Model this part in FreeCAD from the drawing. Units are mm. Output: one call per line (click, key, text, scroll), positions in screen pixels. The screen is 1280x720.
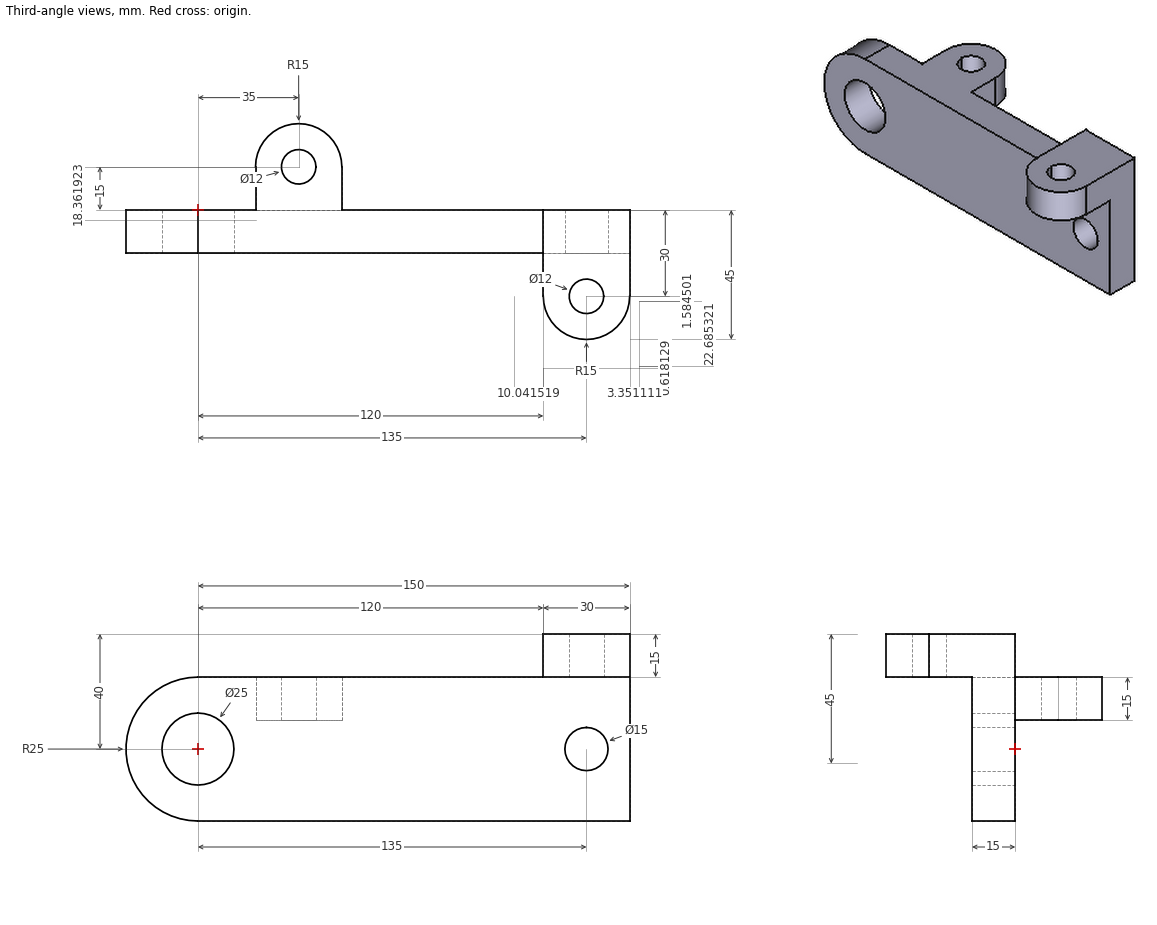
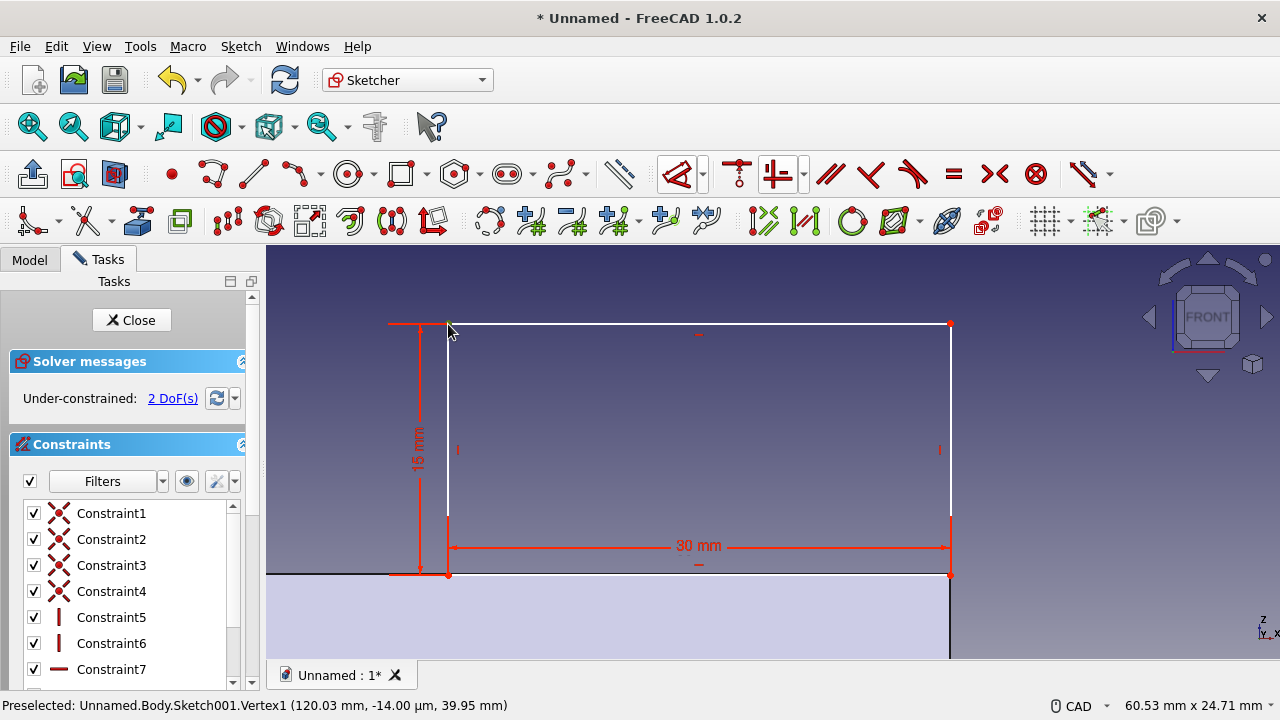
key(i)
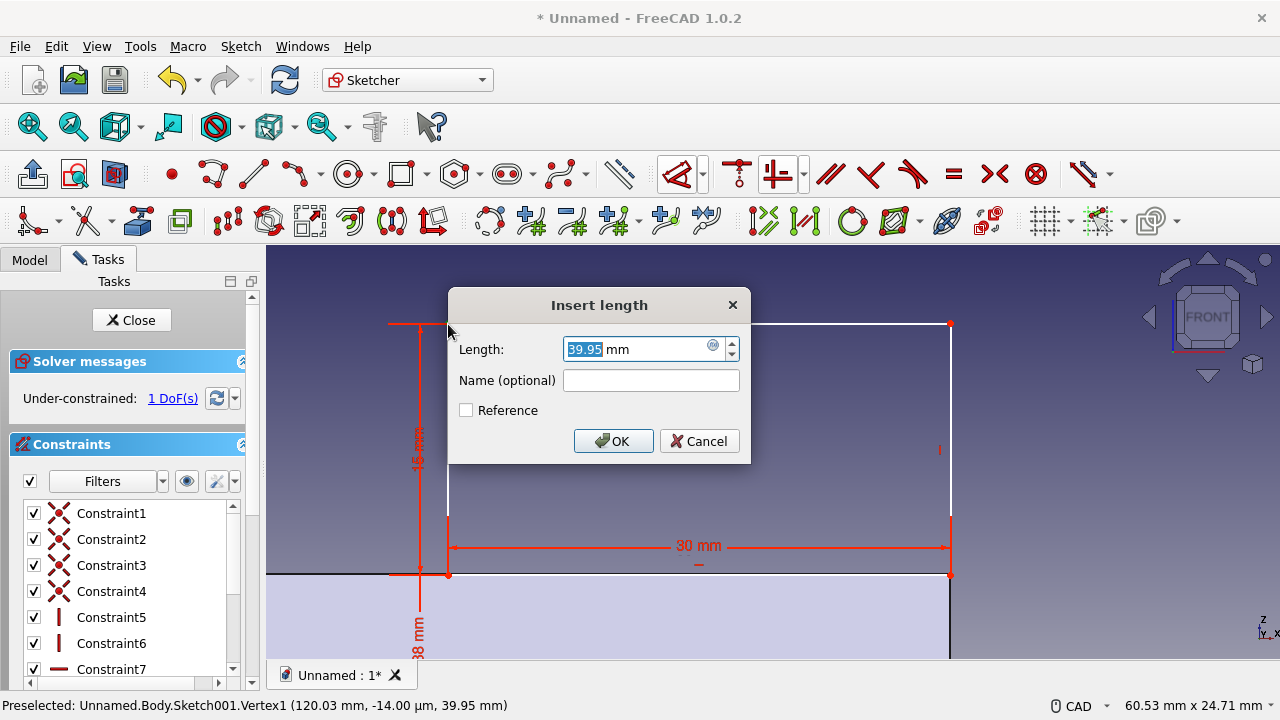
text(40)
key(Return)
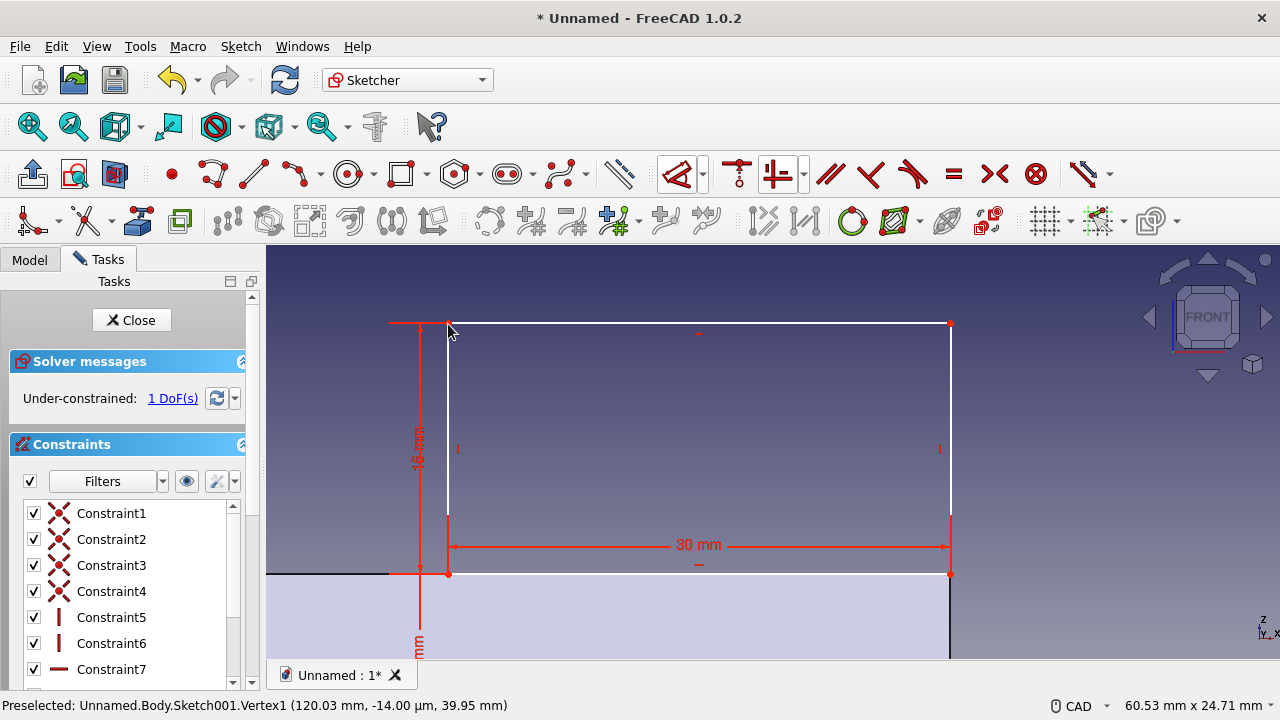
click(448, 323)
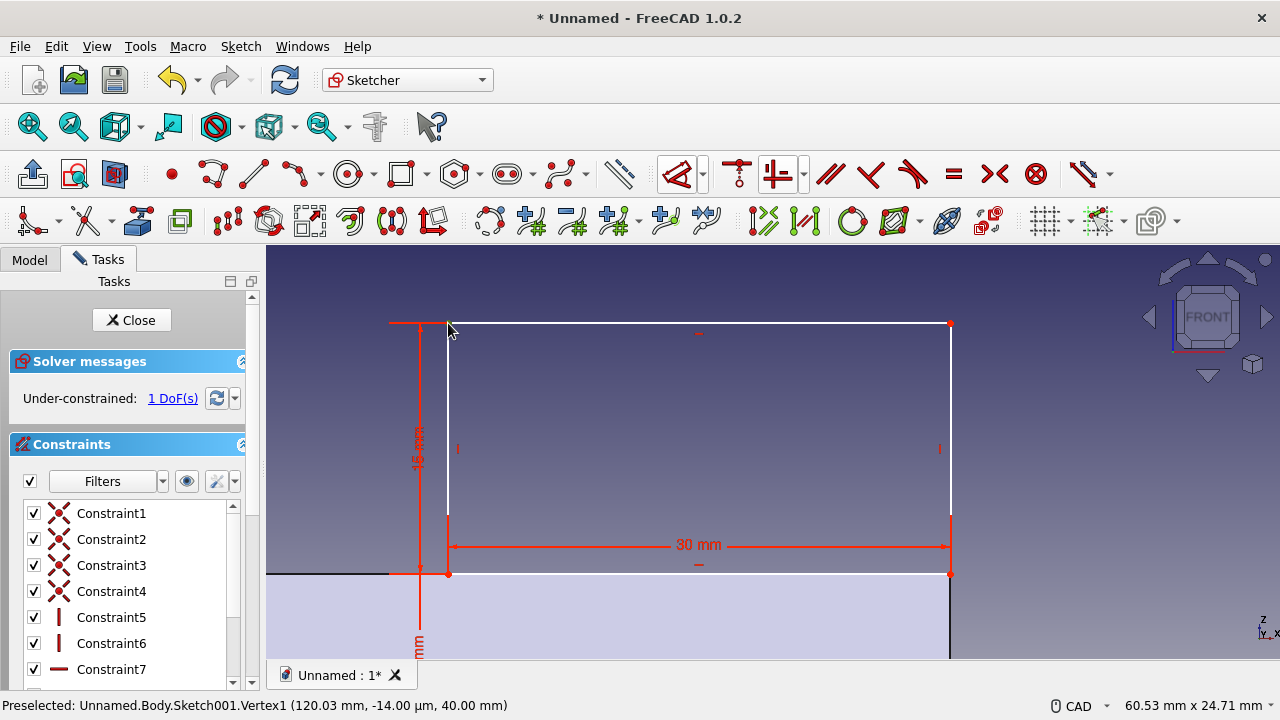
key(l)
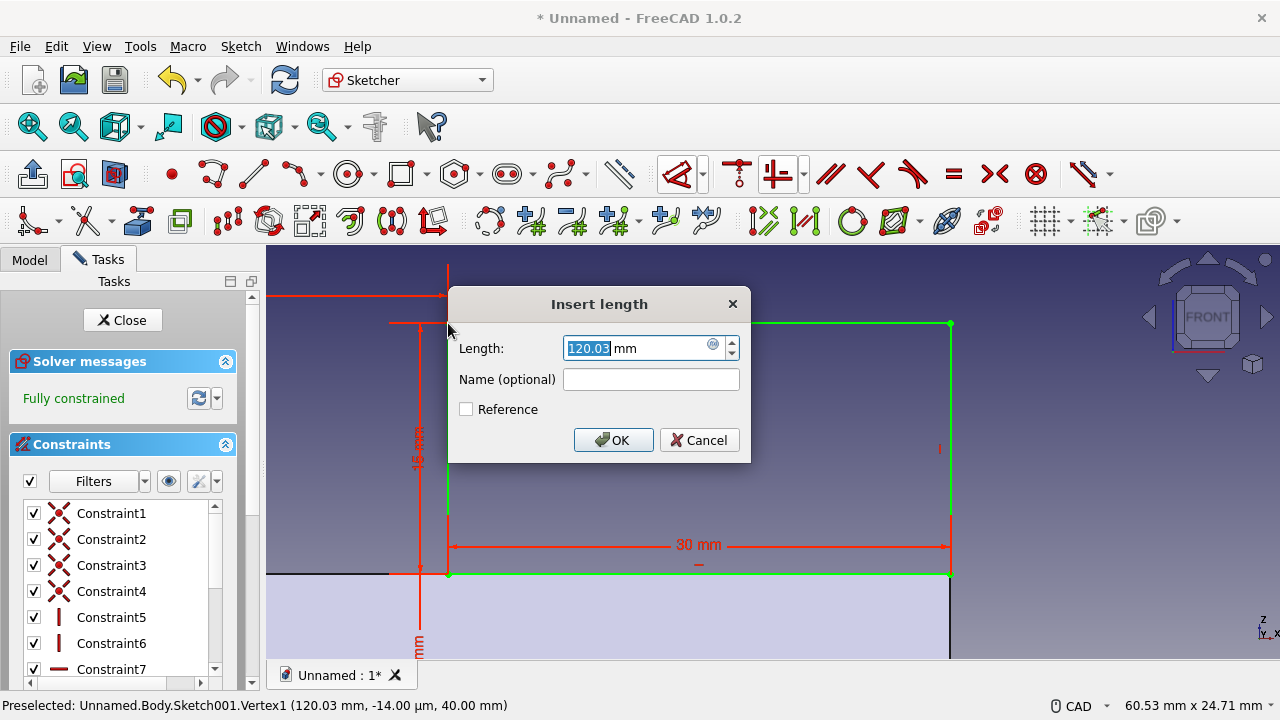
text(120)
key(Return)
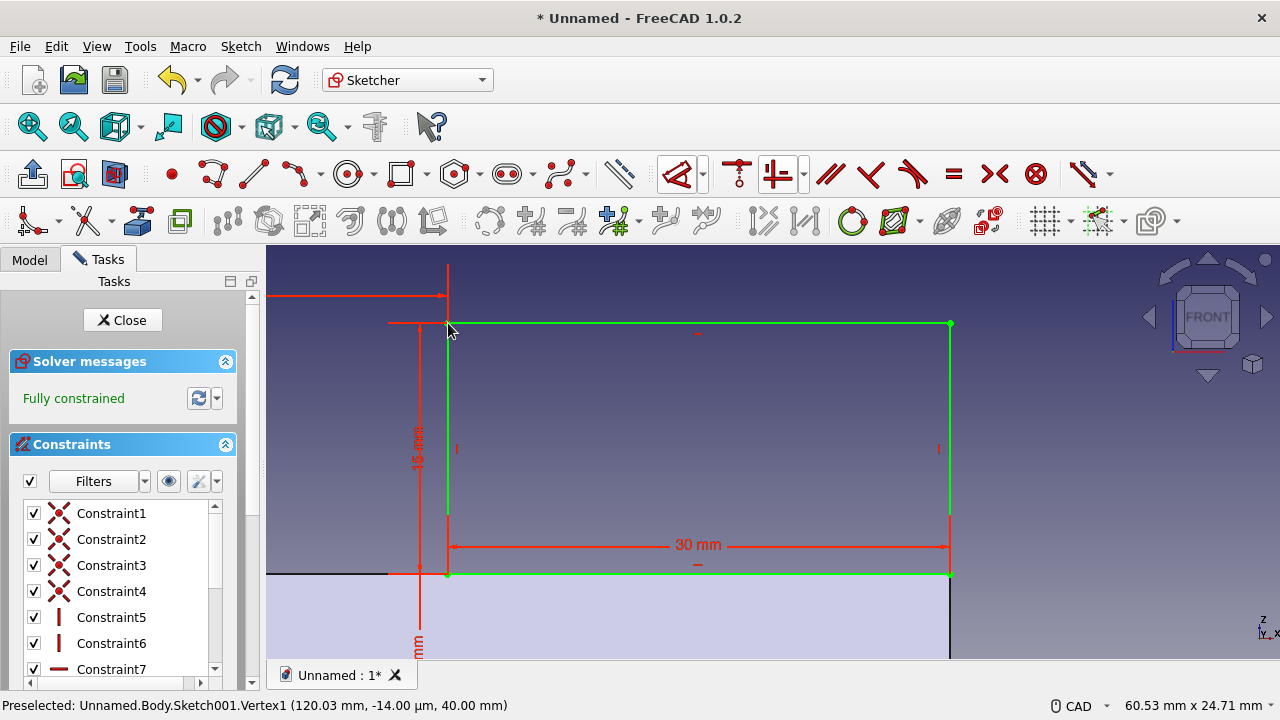
click(123, 320)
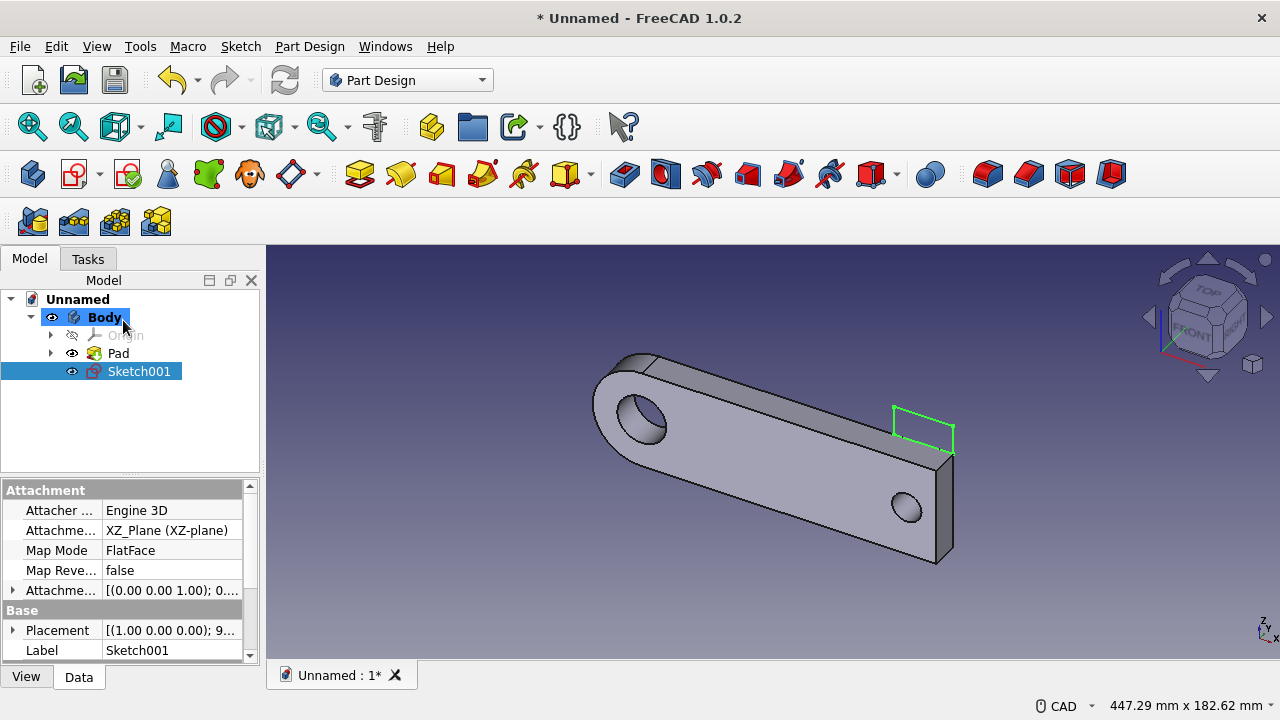
click(360, 174)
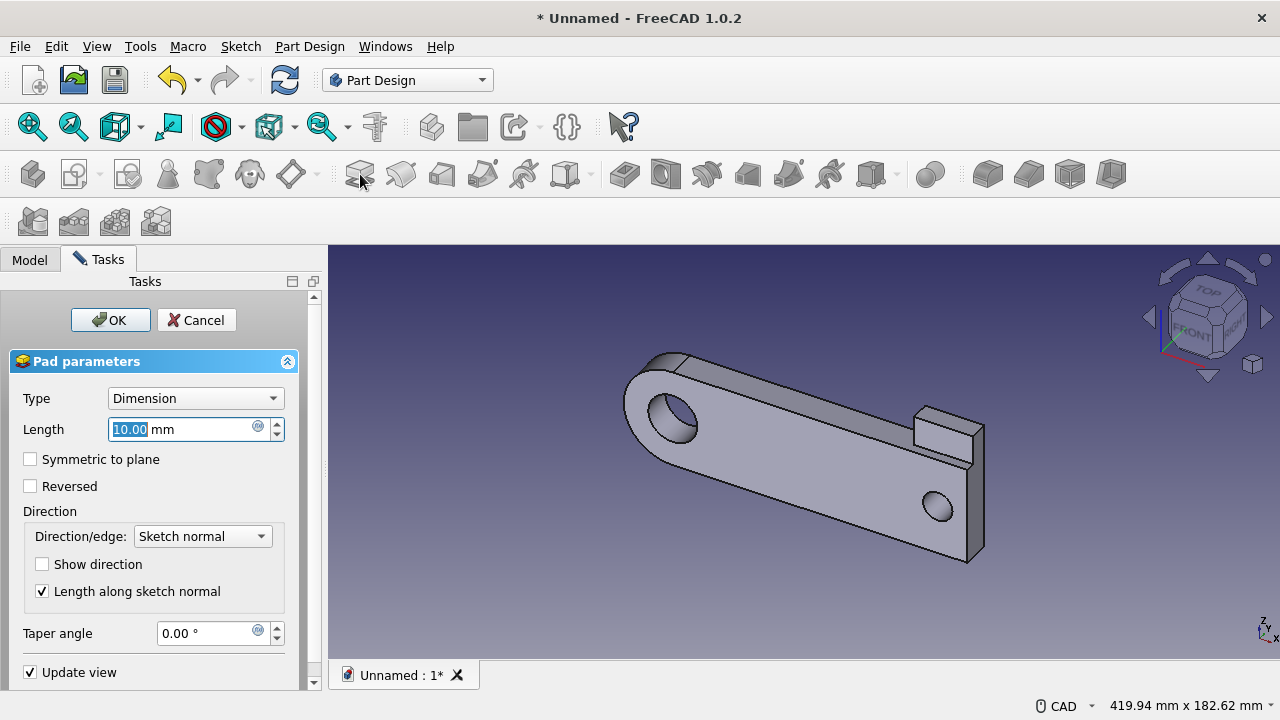
text(45)
key(Tab)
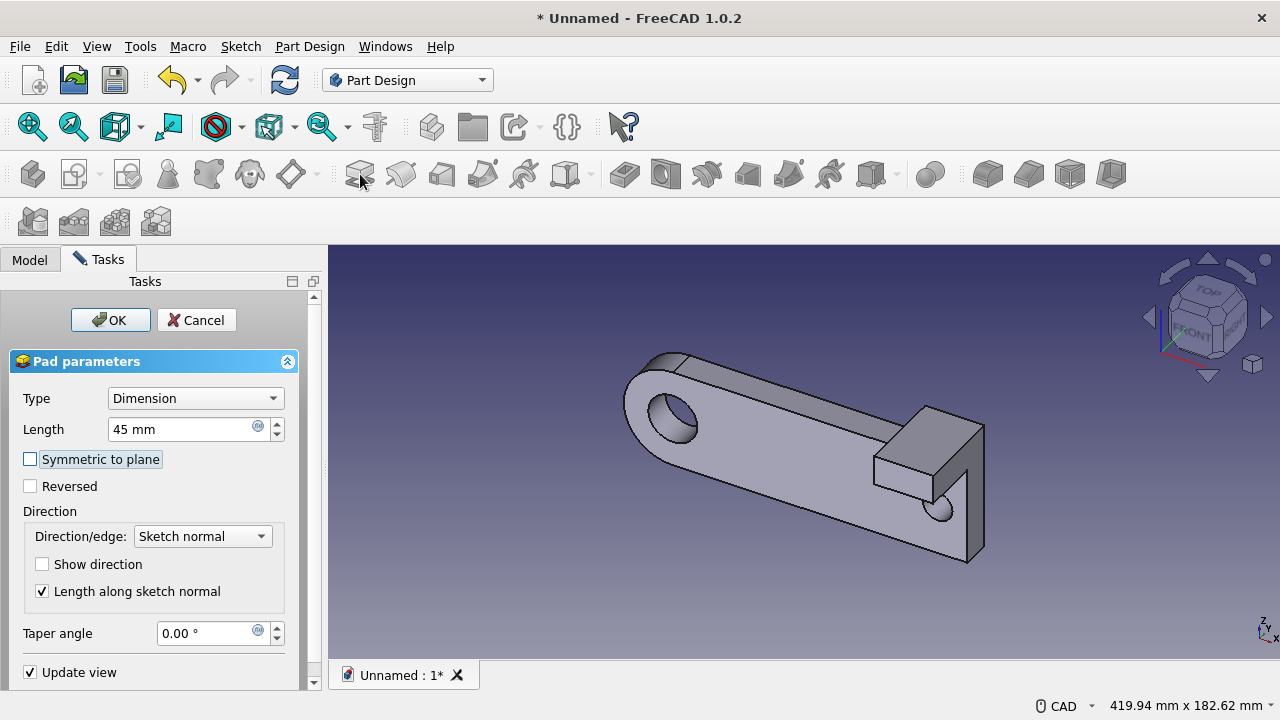
click(111, 320)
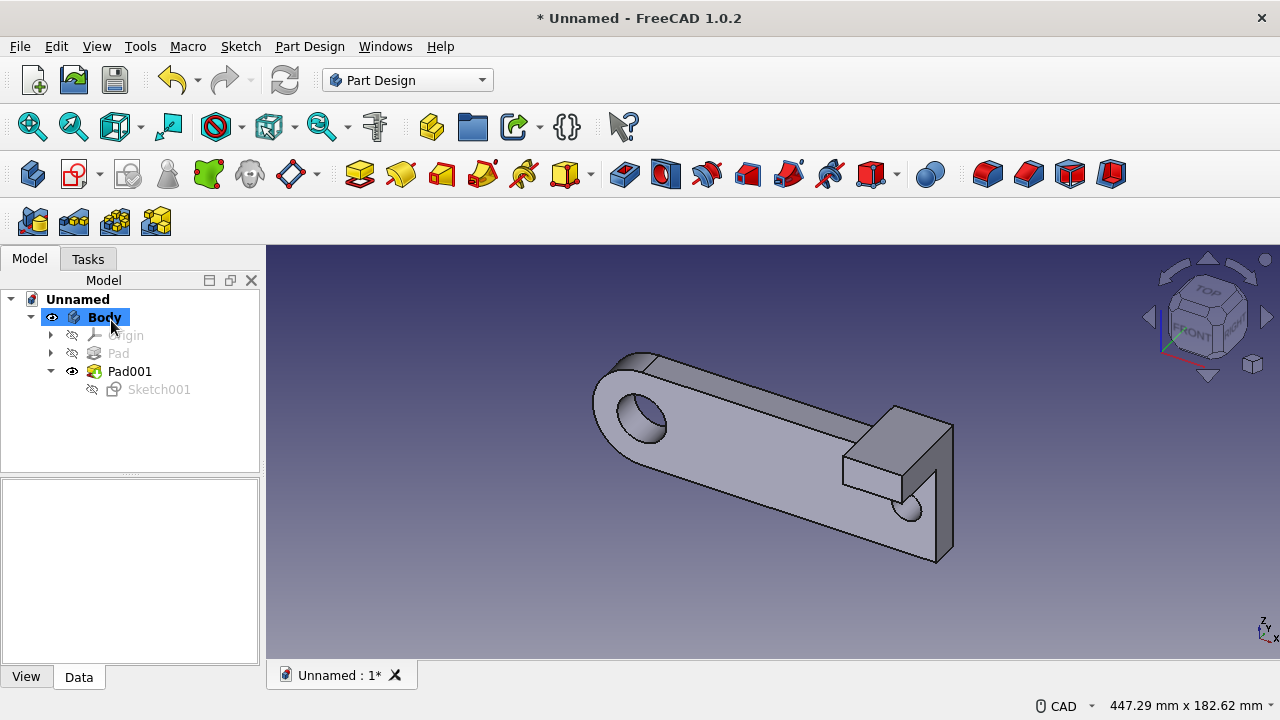
click(906, 432)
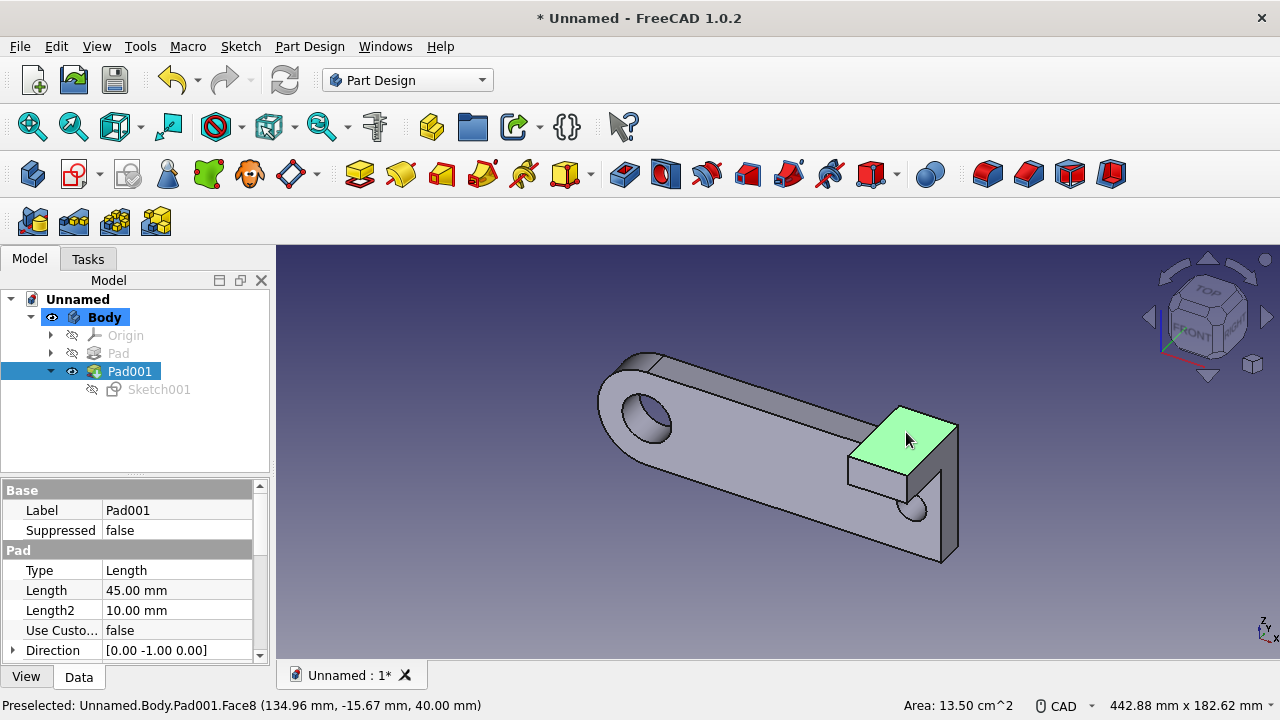
click(74, 174)